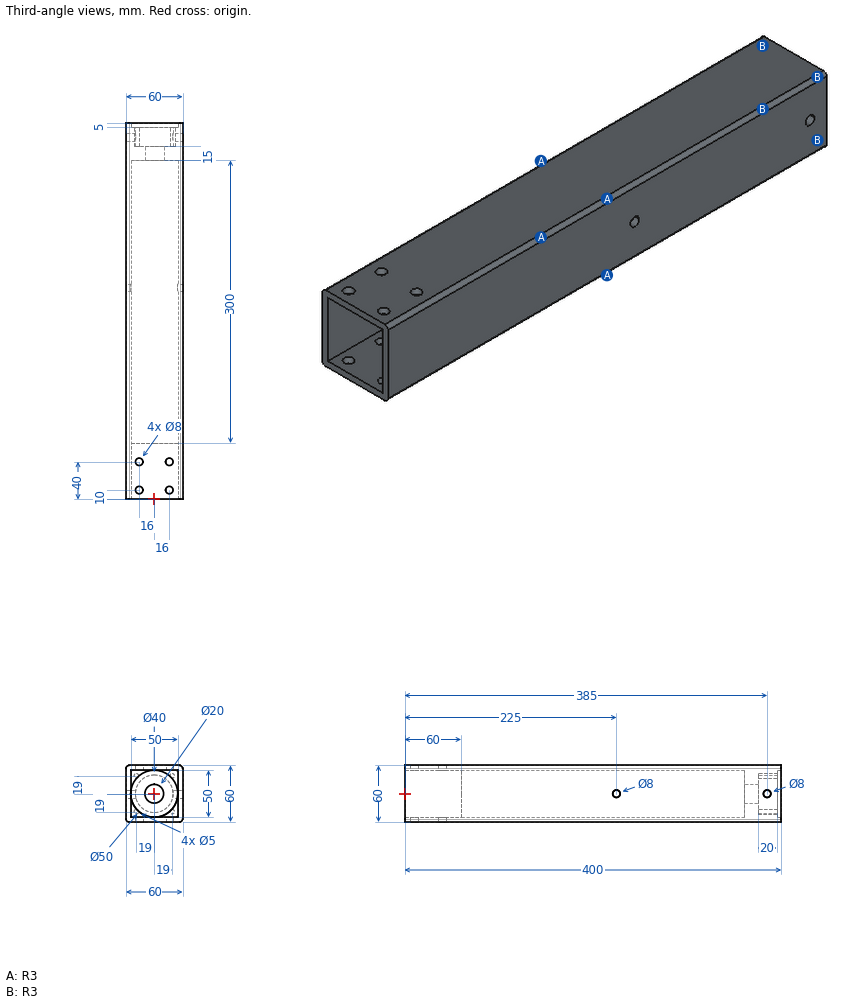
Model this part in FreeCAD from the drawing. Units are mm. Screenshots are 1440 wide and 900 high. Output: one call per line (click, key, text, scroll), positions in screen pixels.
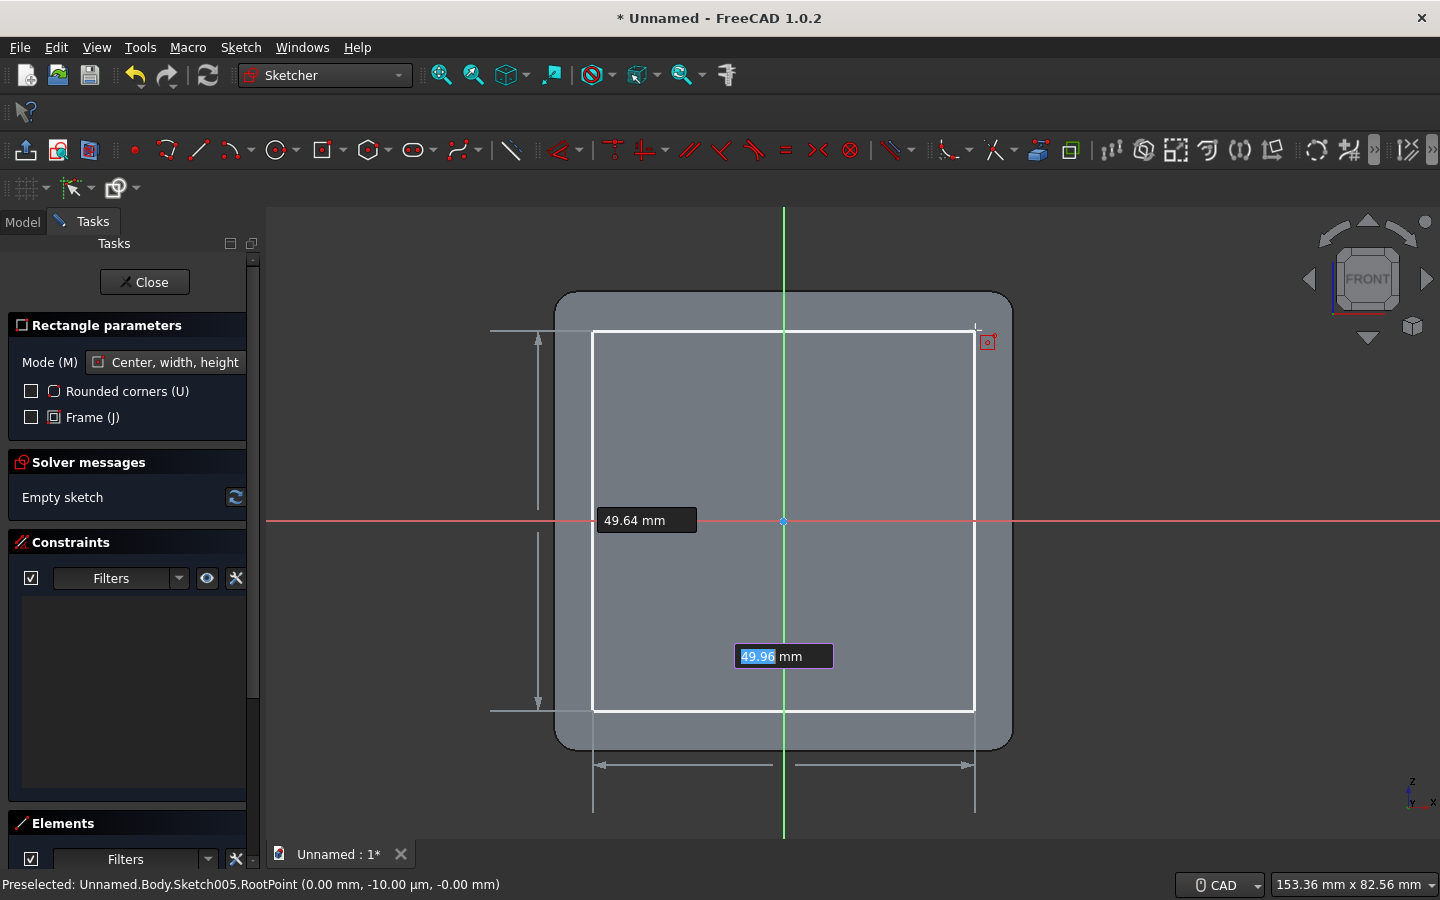
text(50)
key(Tab)
text(50)
key(Return)
key(Escape)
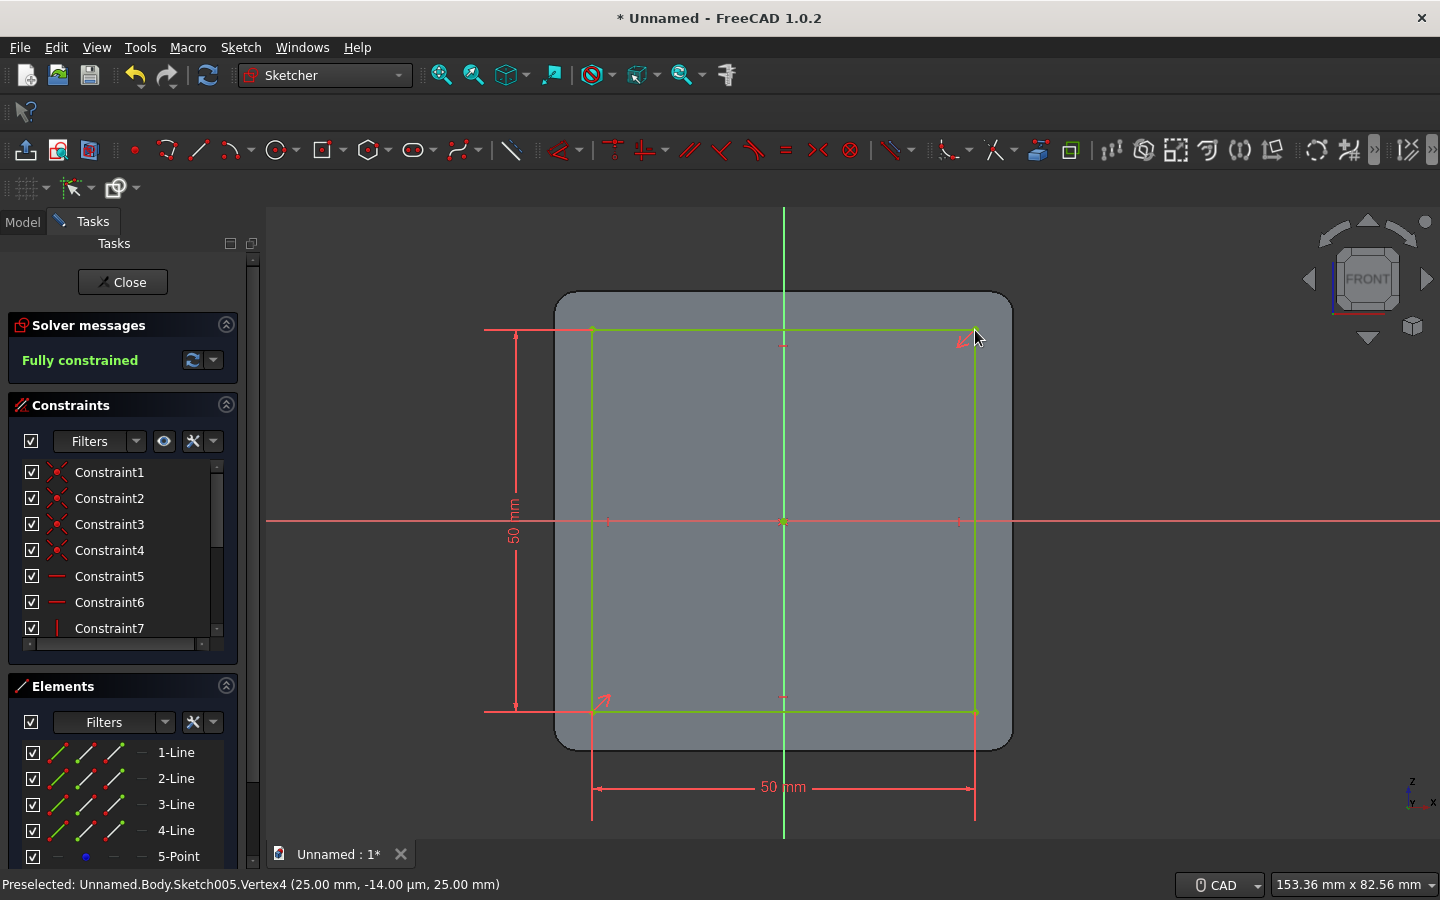
click(123, 282)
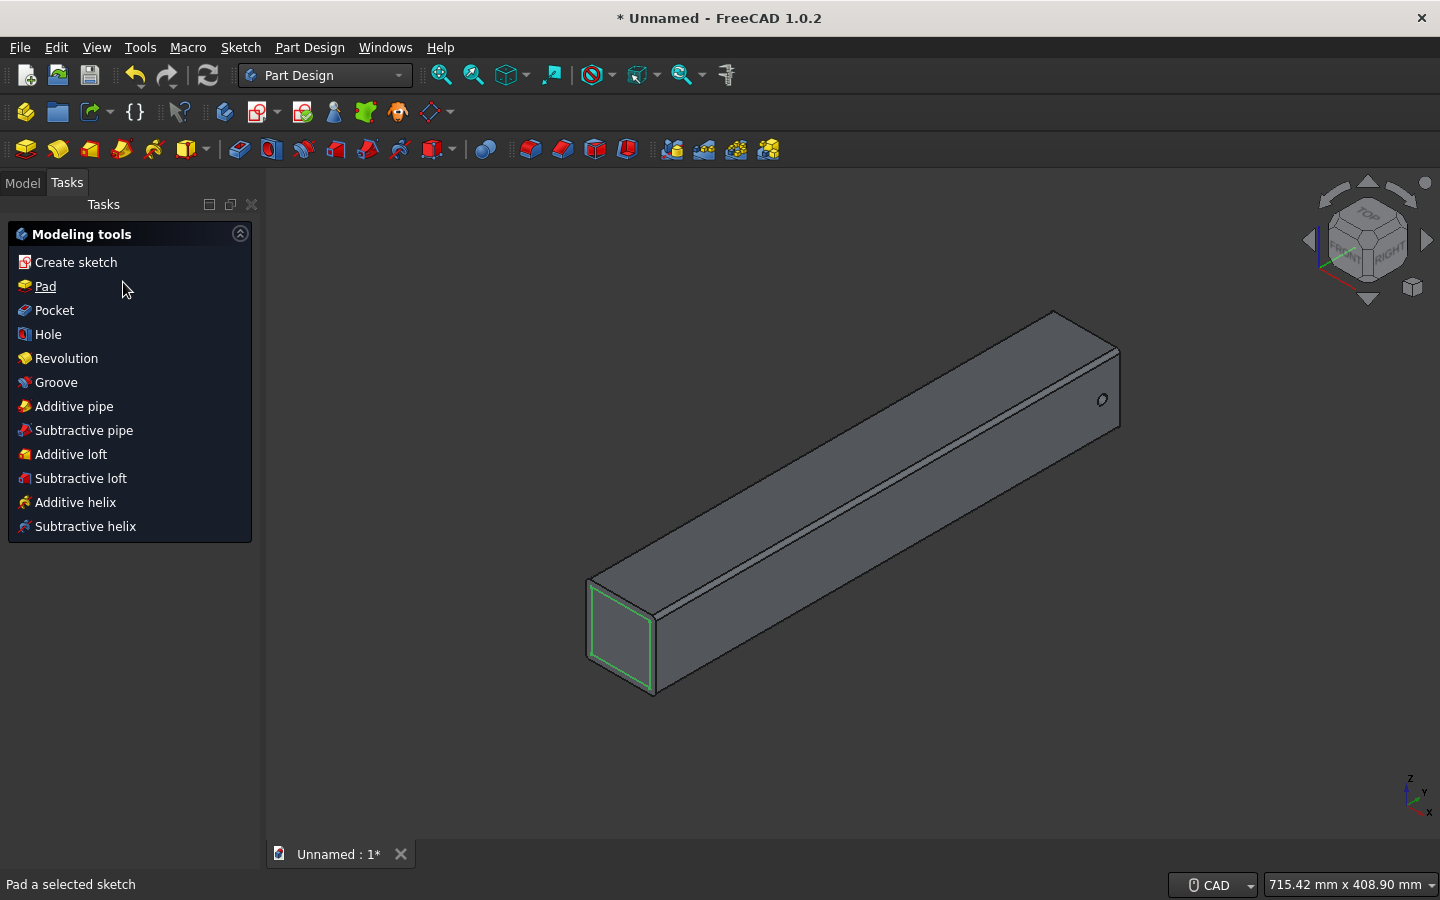
click(240, 150)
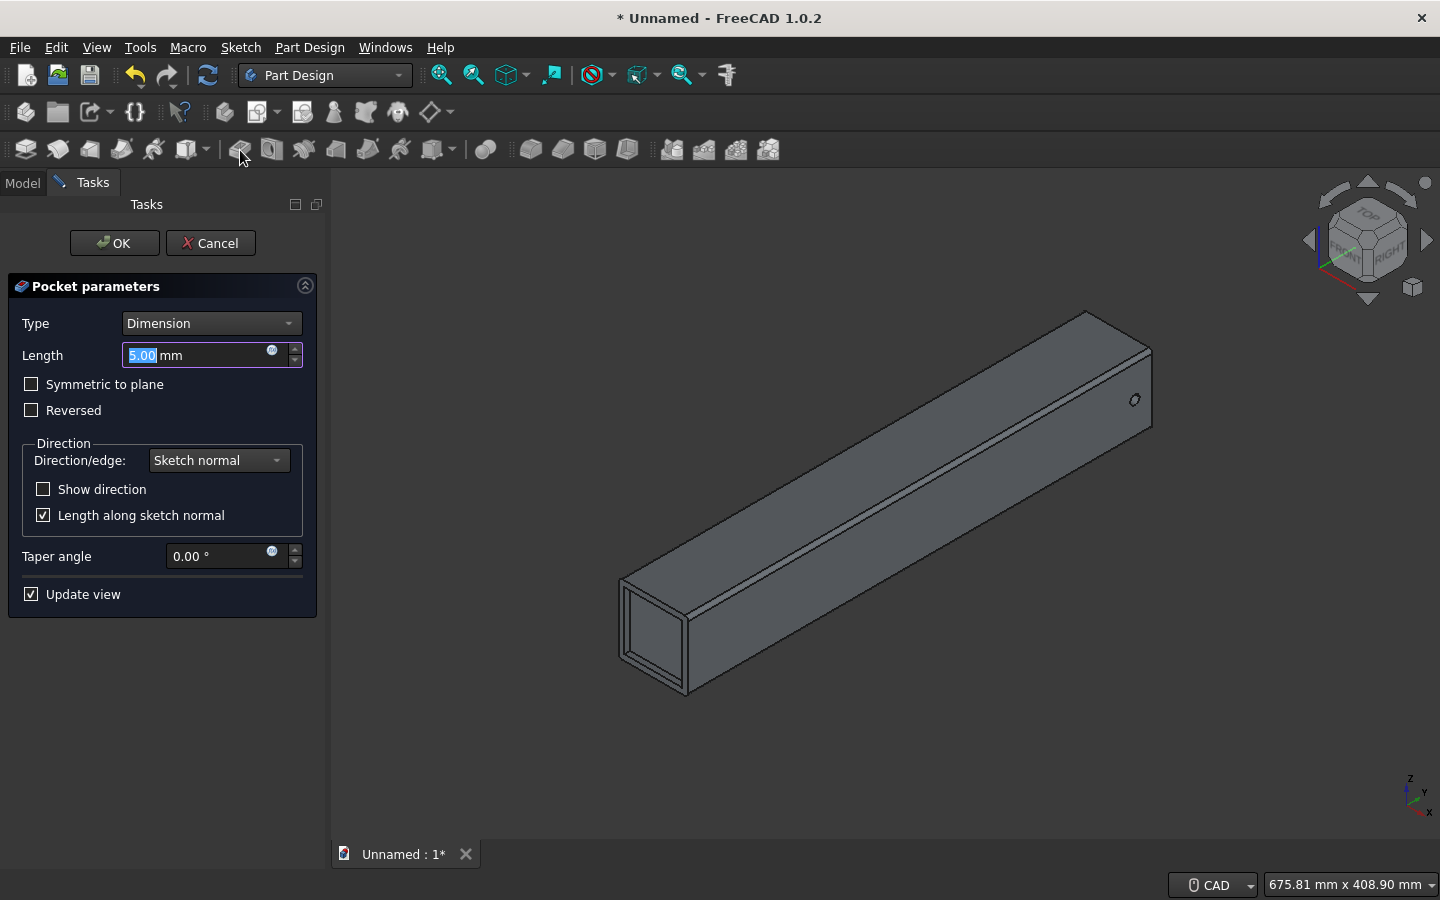
text(60)
key(Tab)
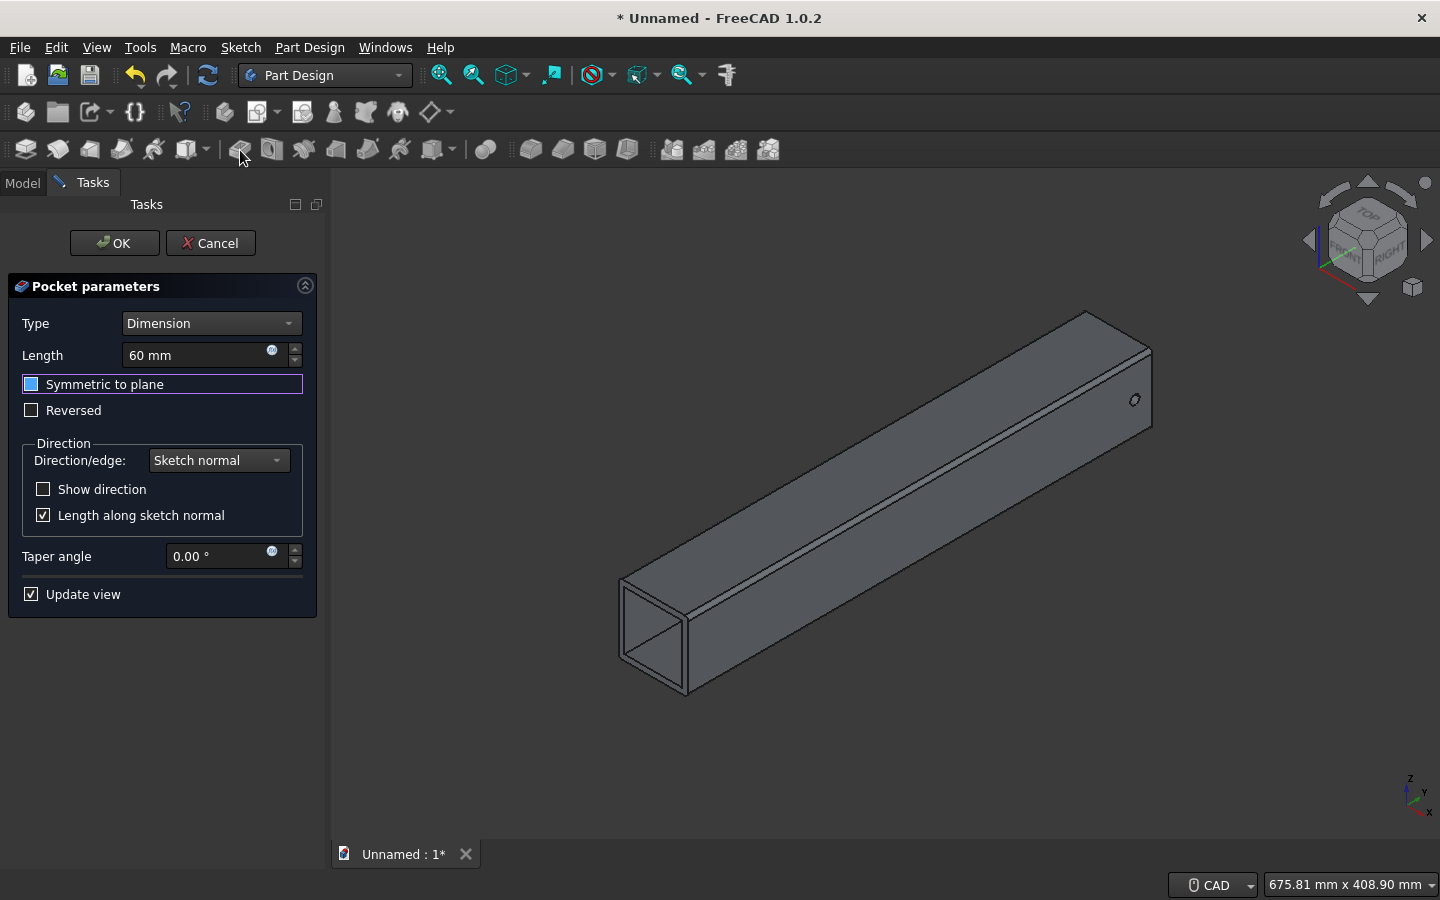
click(115, 243)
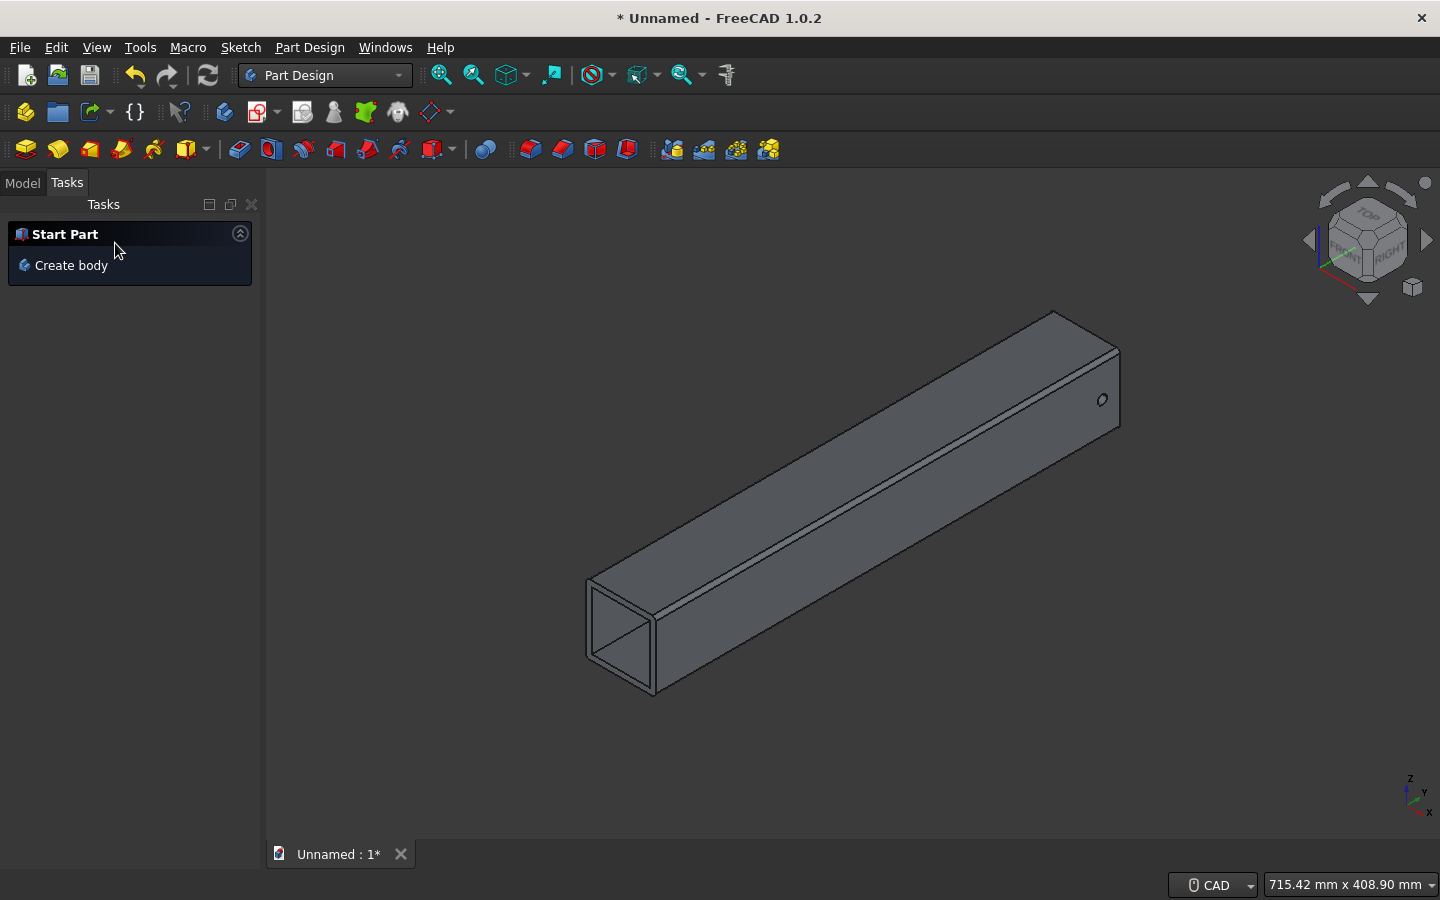
key(1)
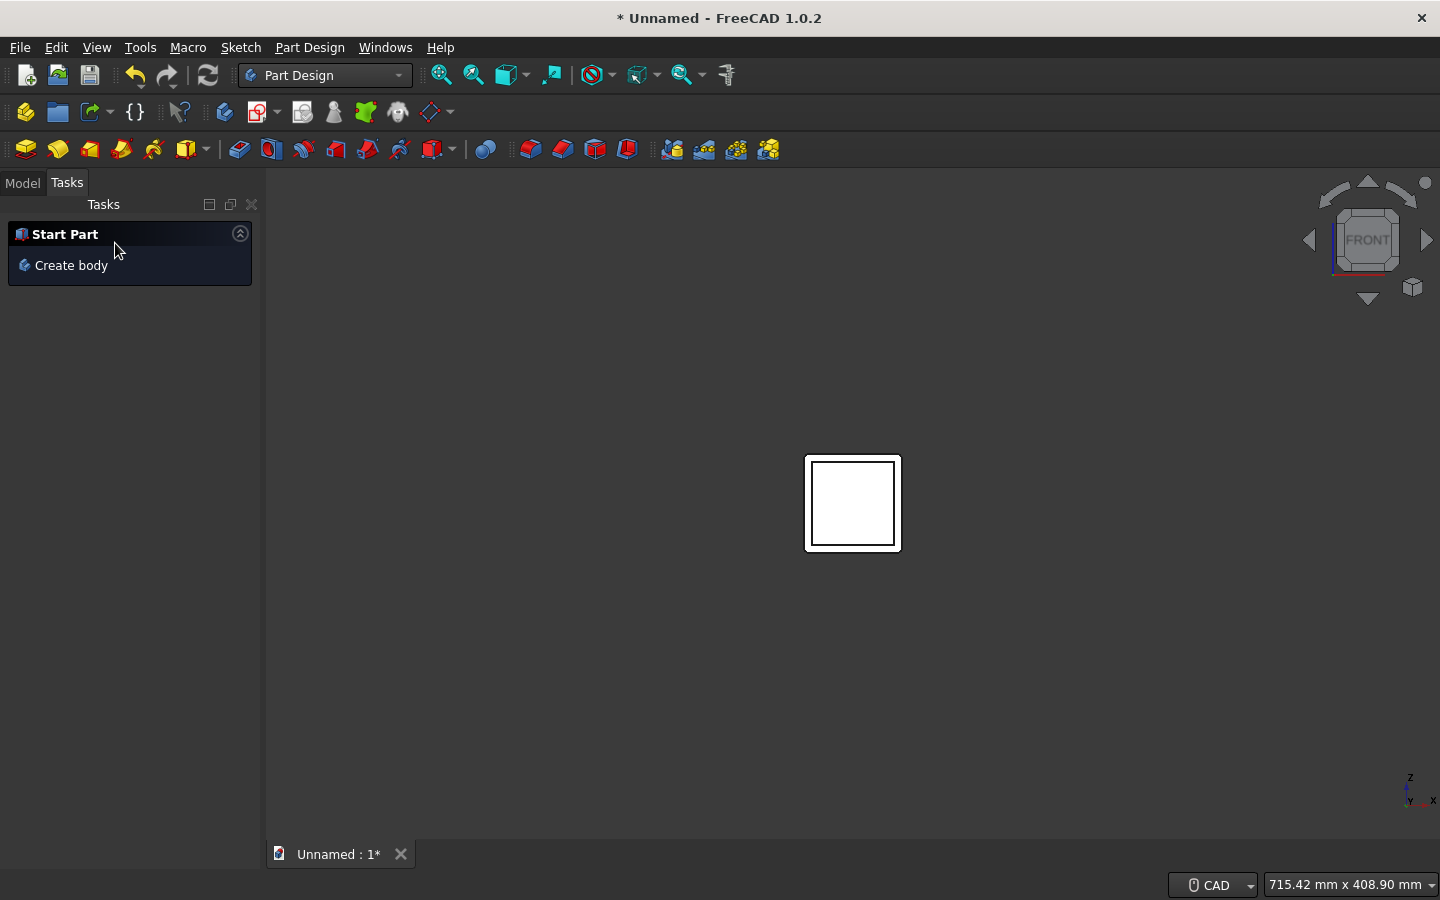
click(442, 76)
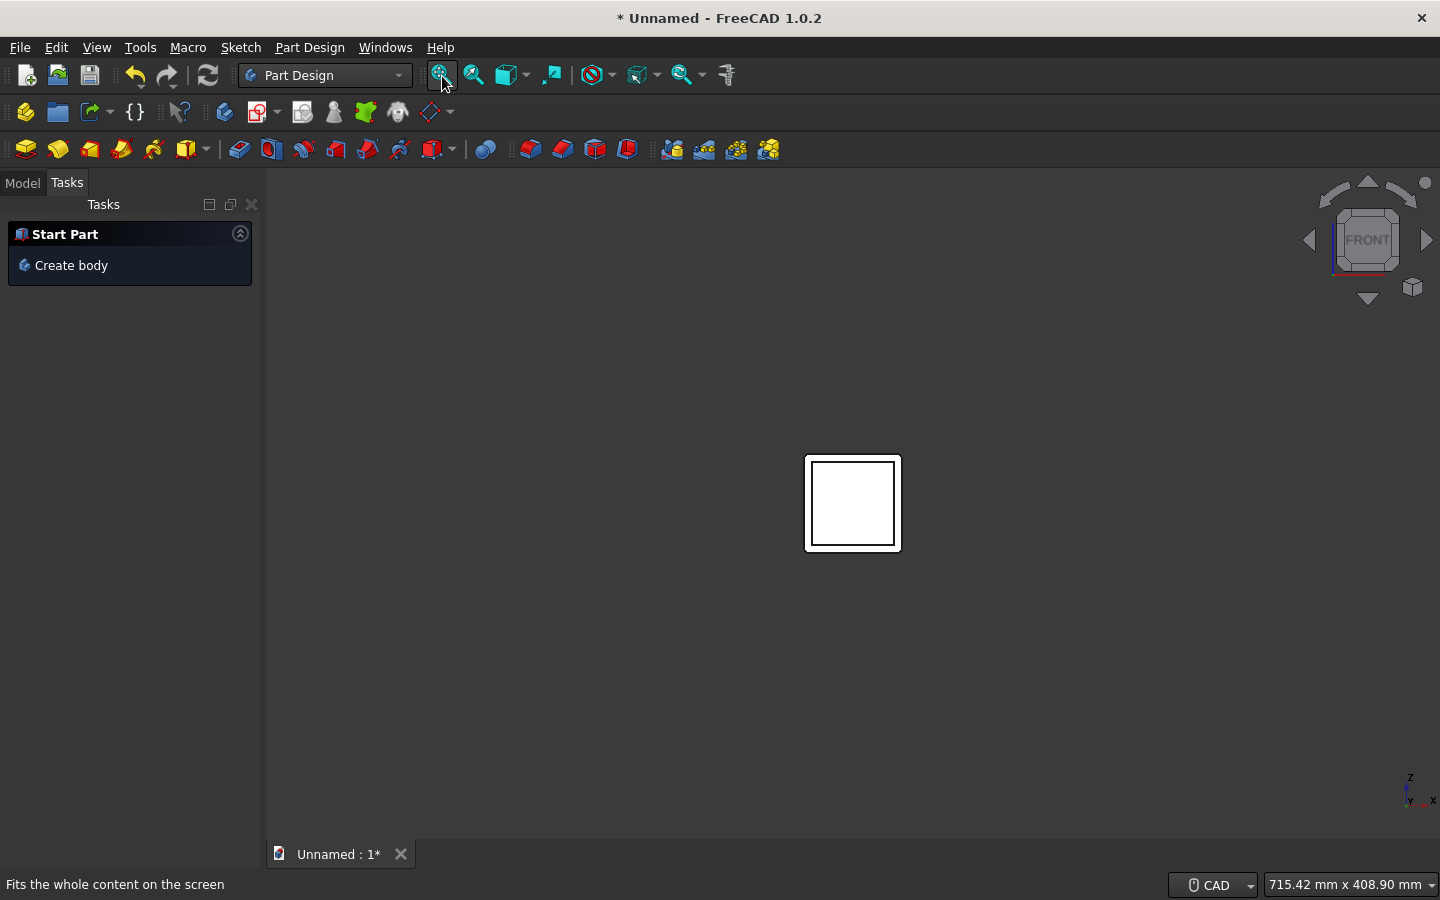
click(853, 503)